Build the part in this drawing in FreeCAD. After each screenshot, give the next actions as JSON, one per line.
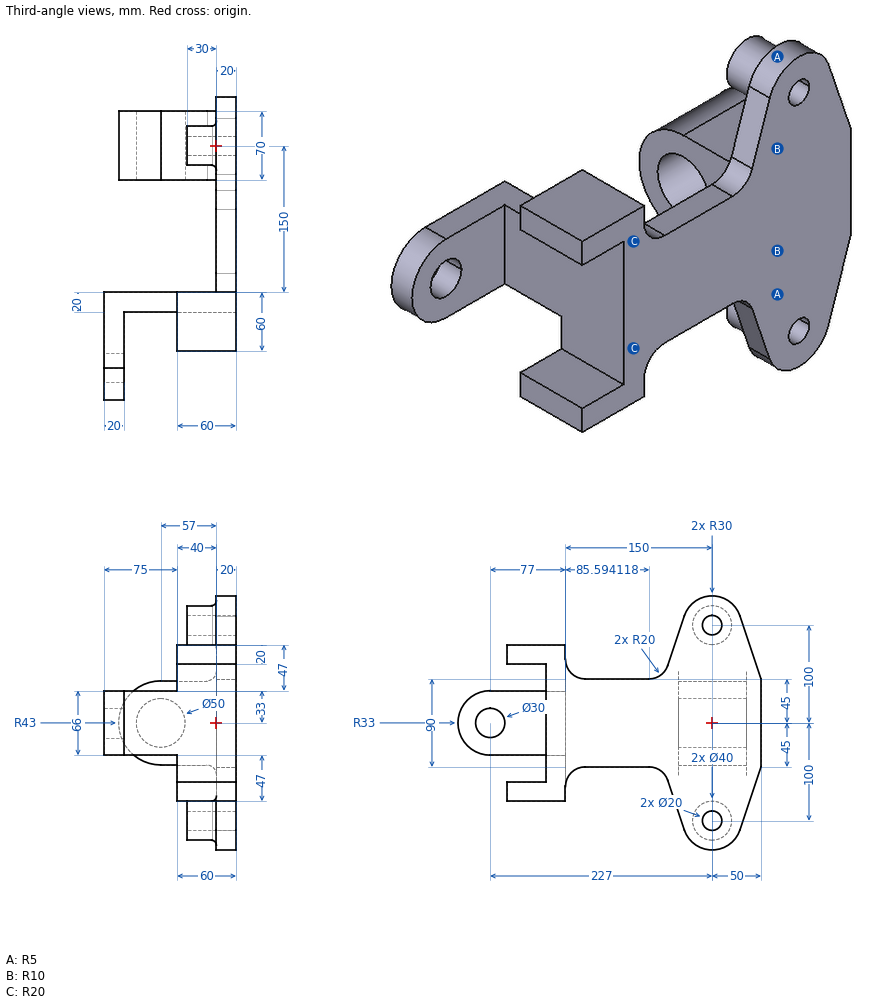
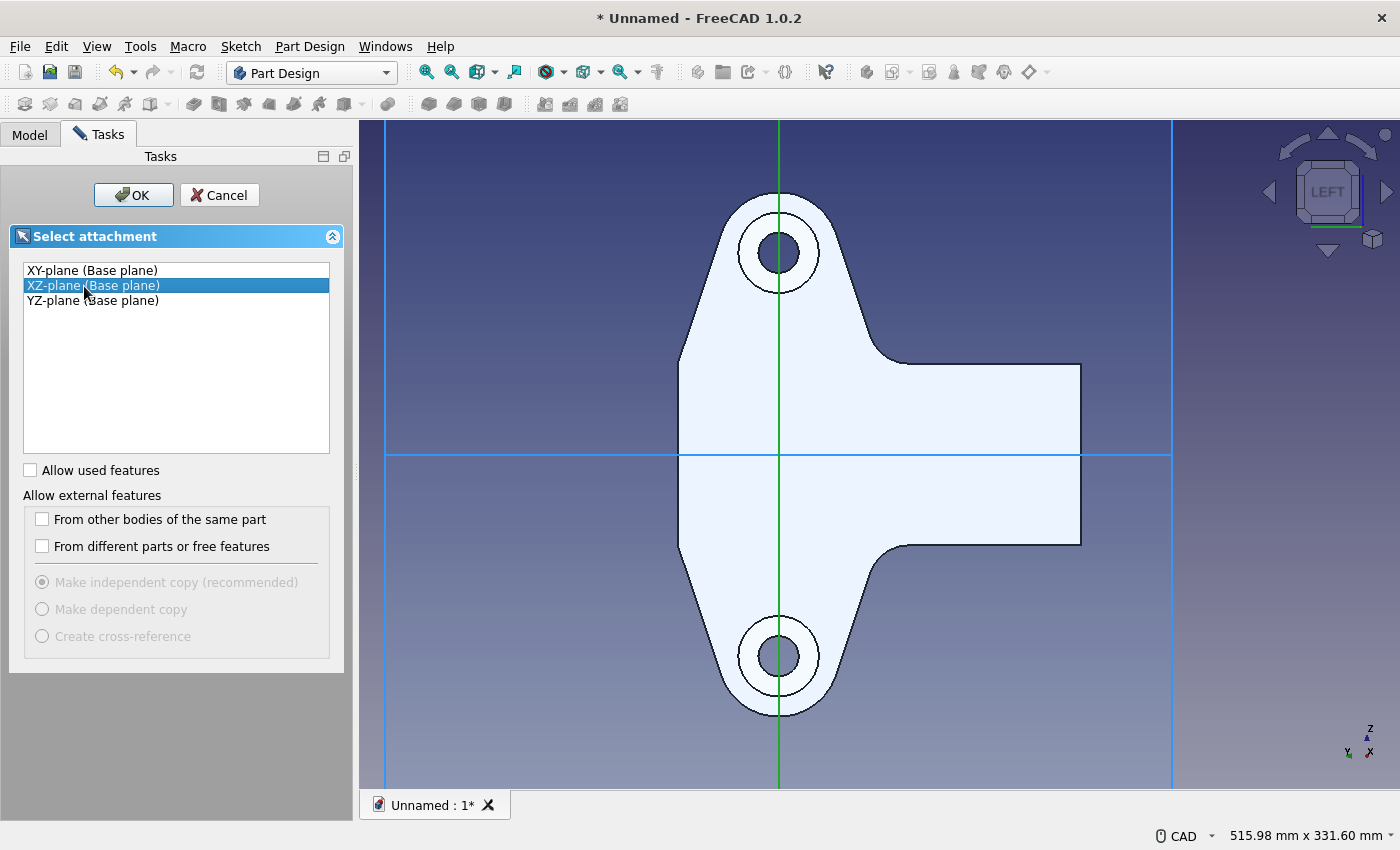
{"action": "left_click", "coordinate": [134, 195]}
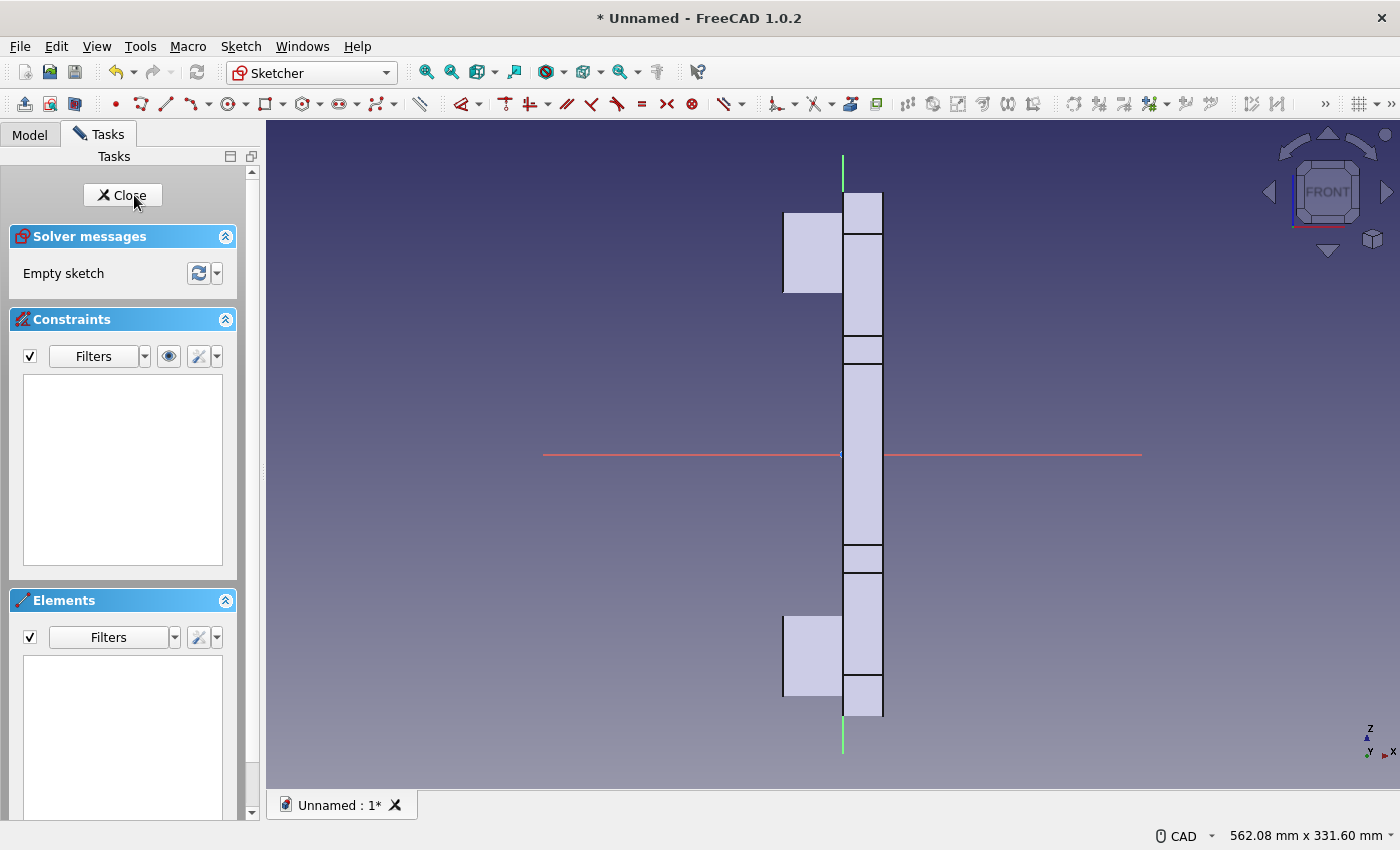
{"action": "left_click", "coordinate": [75, 104]}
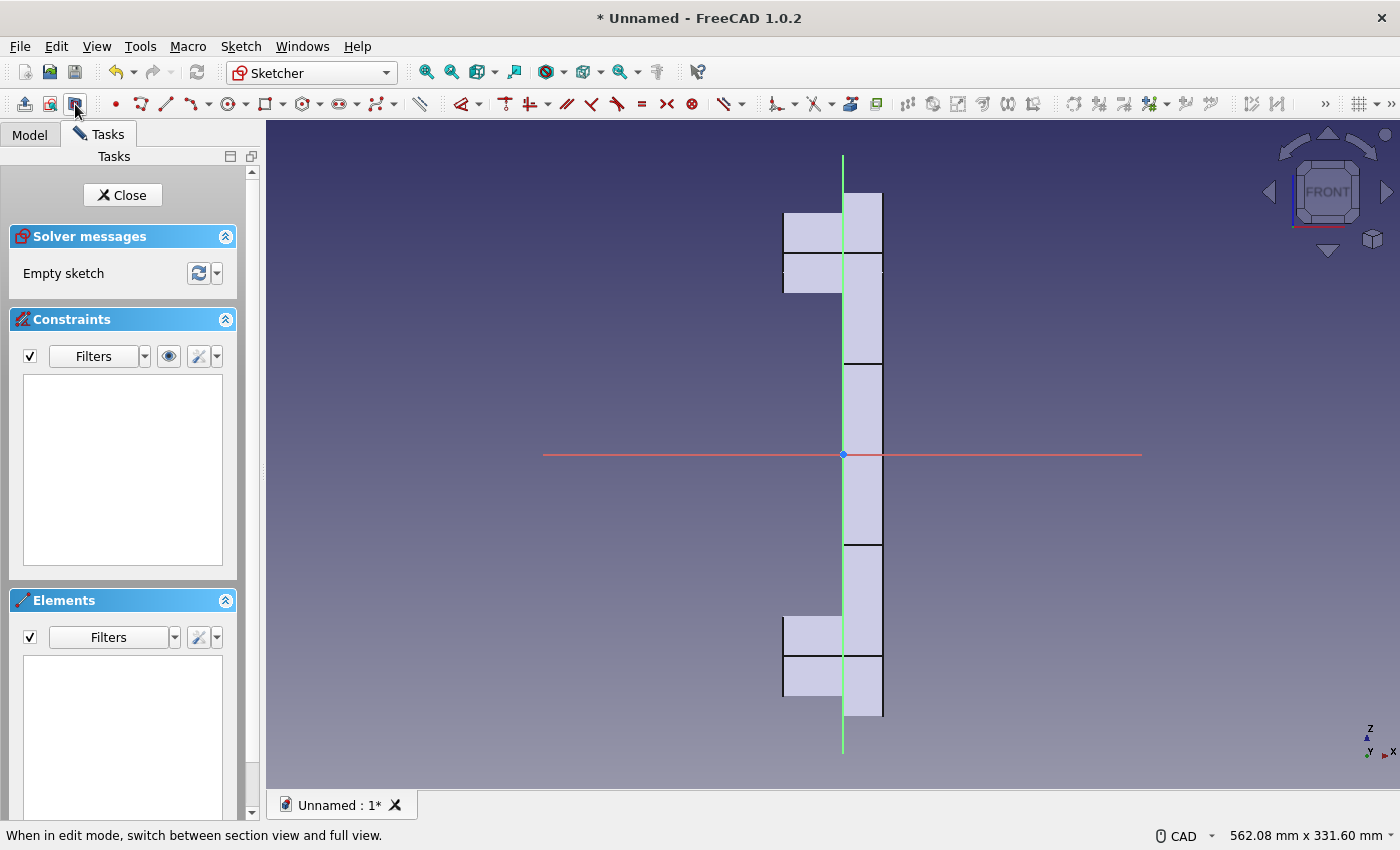
{"action": "scroll", "coordinate": [729, 455], "scroll_direction": "up", "scroll_amount": 5}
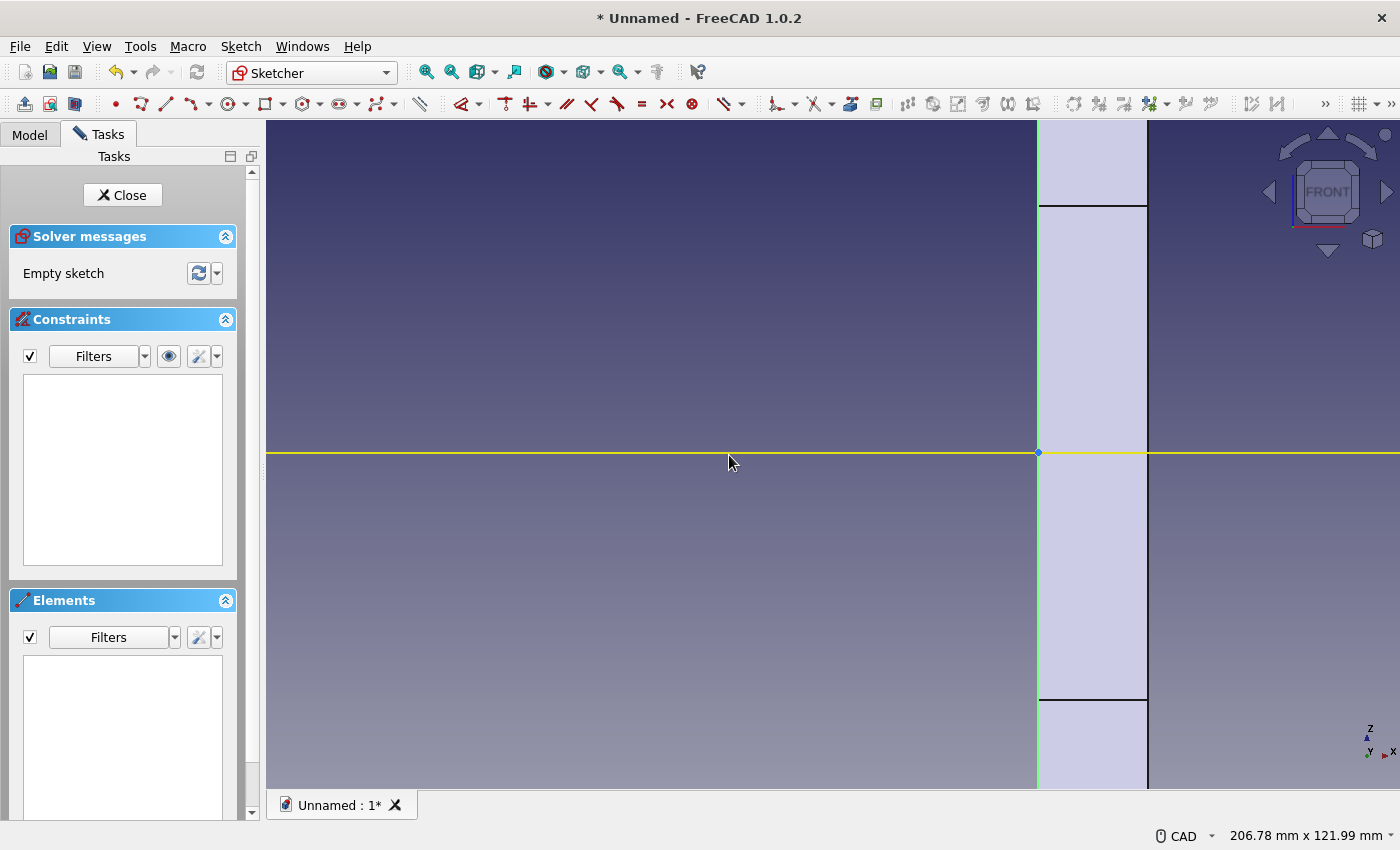
{"action": "key", "text": "g m"}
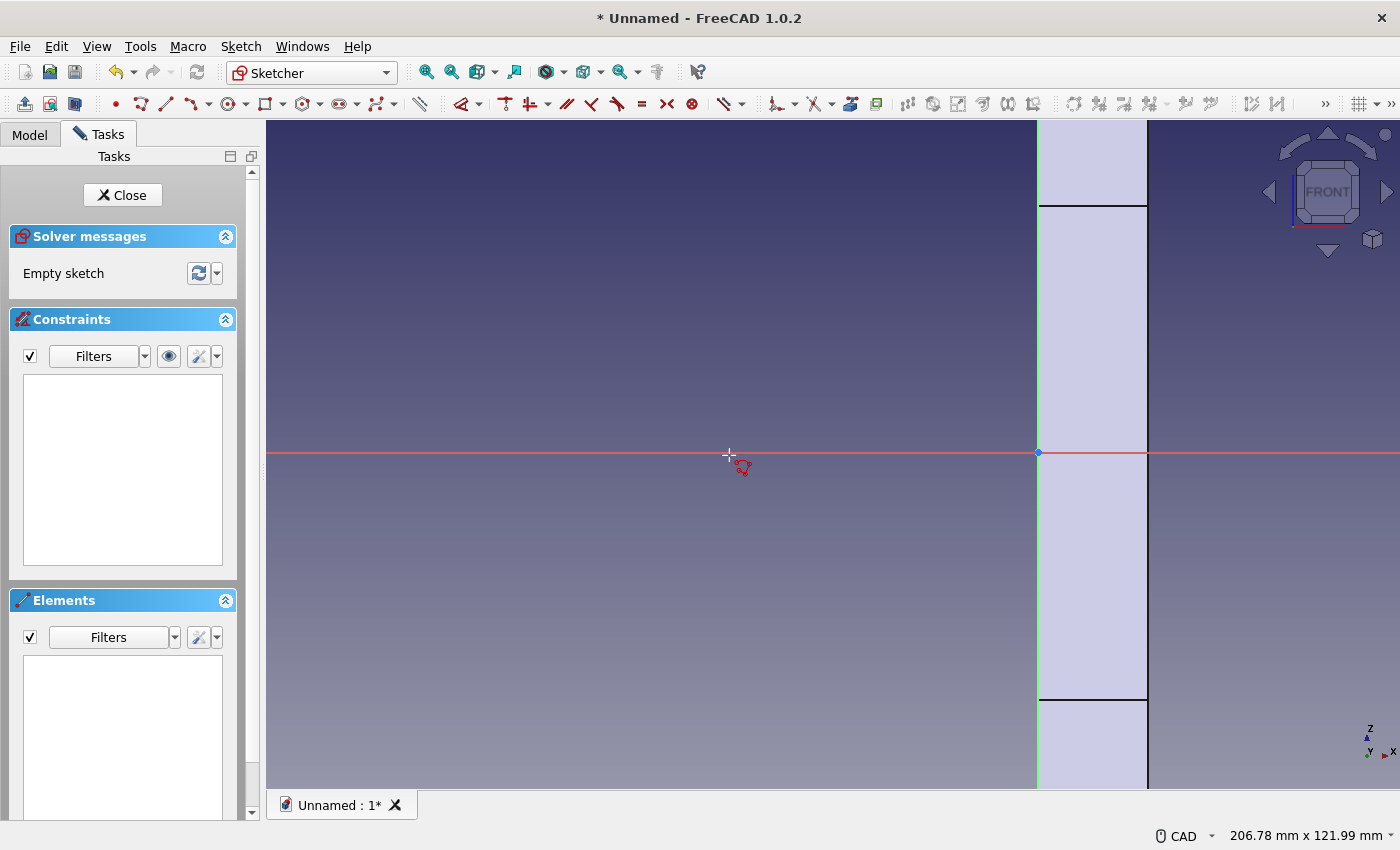
{"action": "left_click", "coordinate": [726, 217]}
{"action": "left_click", "coordinate": [1038, 217]}
{"action": "left_click", "coordinate": [1029, 689]}
{"action": "left_click", "coordinate": [726, 689]}
{"action": "right_click", "coordinate": [726, 689]}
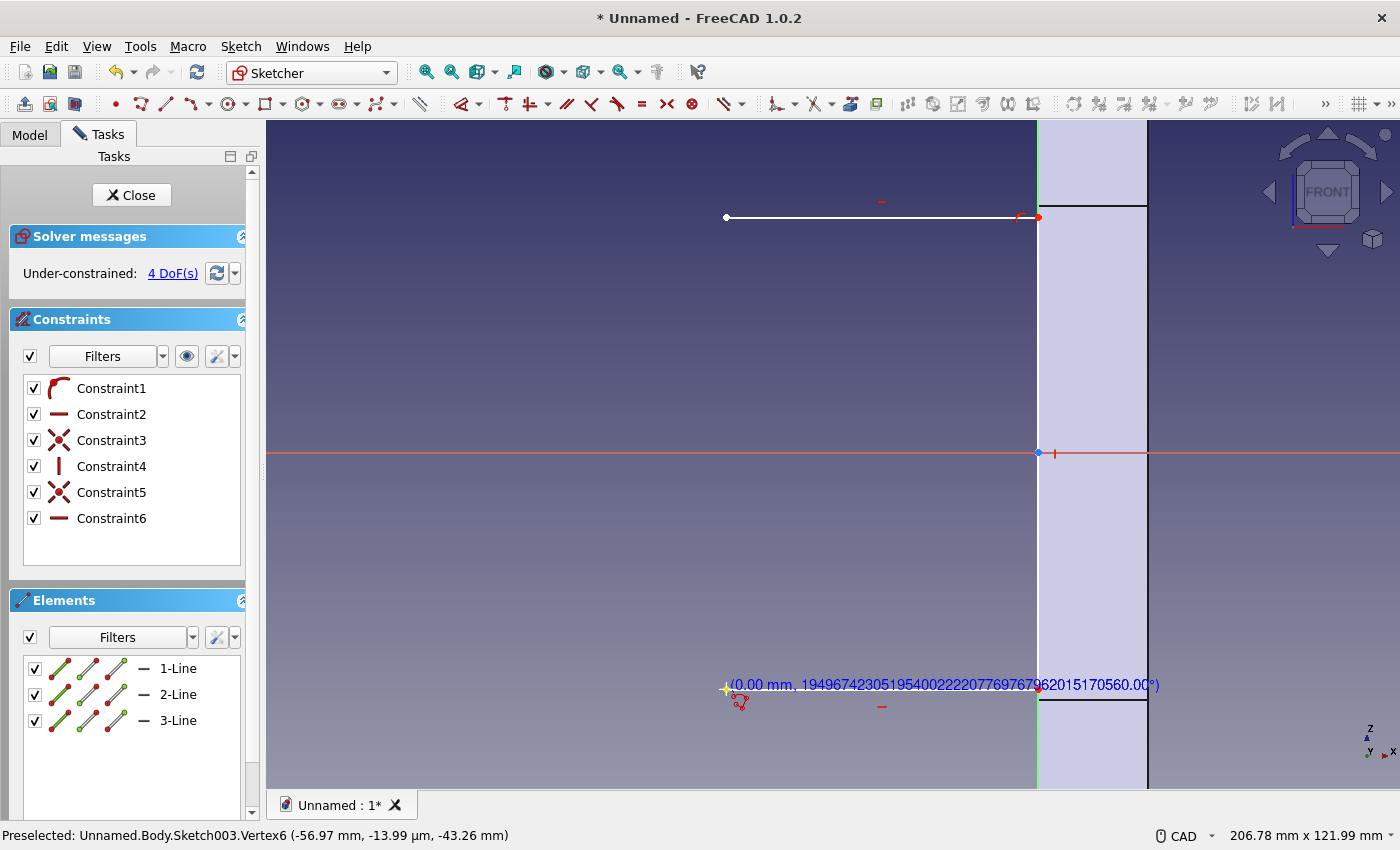
{"action": "left_click", "coordinate": [190, 104]}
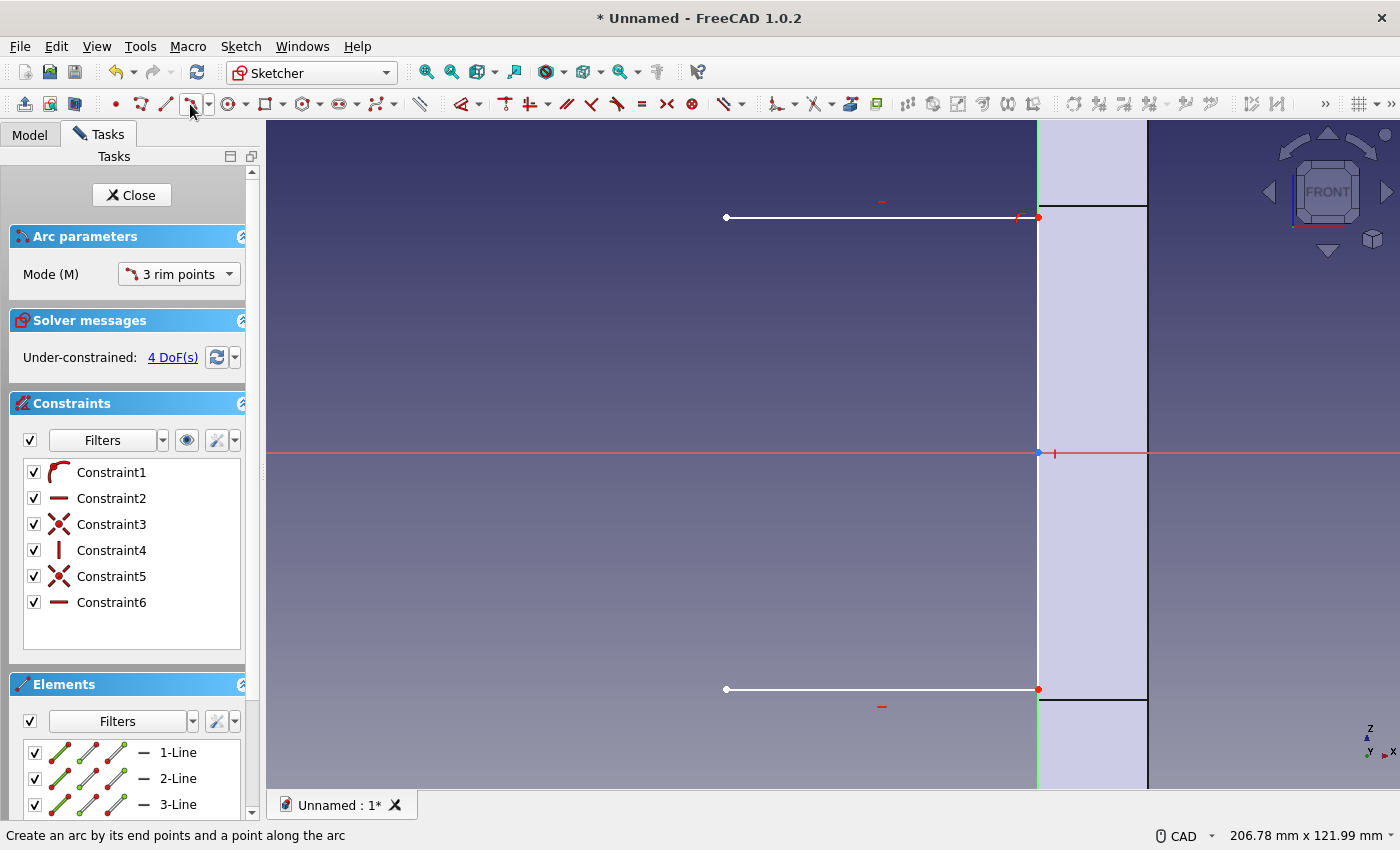
{"action": "left_click", "coordinate": [726, 690]}
{"action": "left_click", "coordinate": [726, 218]}
{"action": "left_click", "coordinate": [502, 380]}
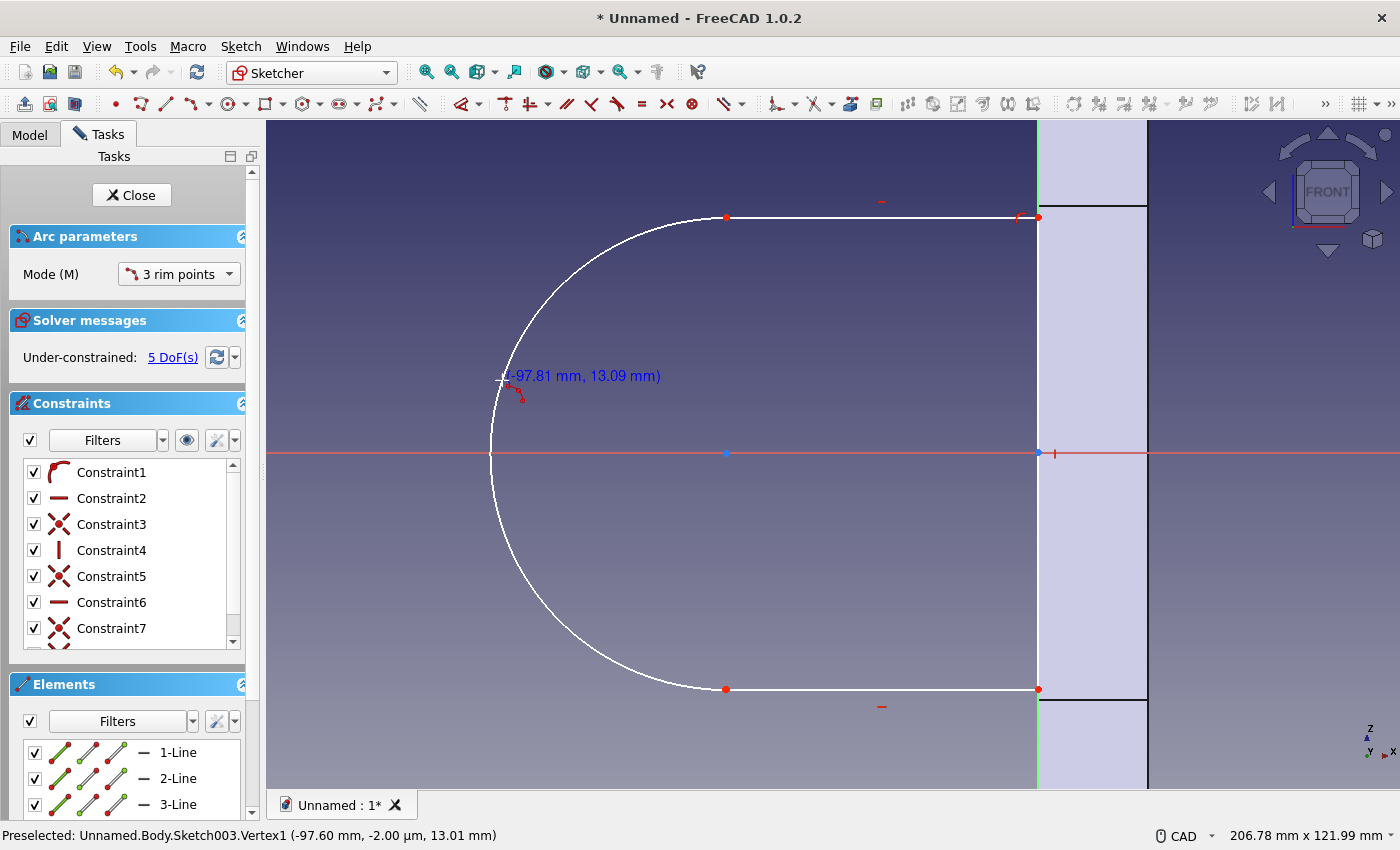
{"action": "left_click", "coordinate": [228, 104]}